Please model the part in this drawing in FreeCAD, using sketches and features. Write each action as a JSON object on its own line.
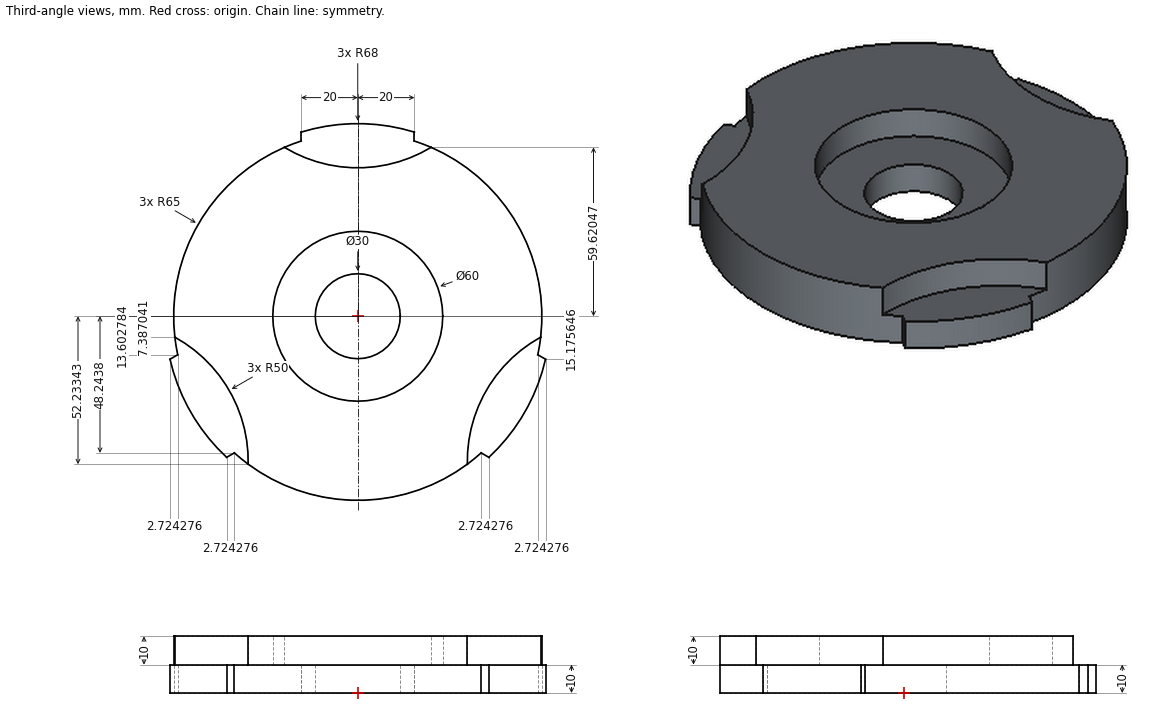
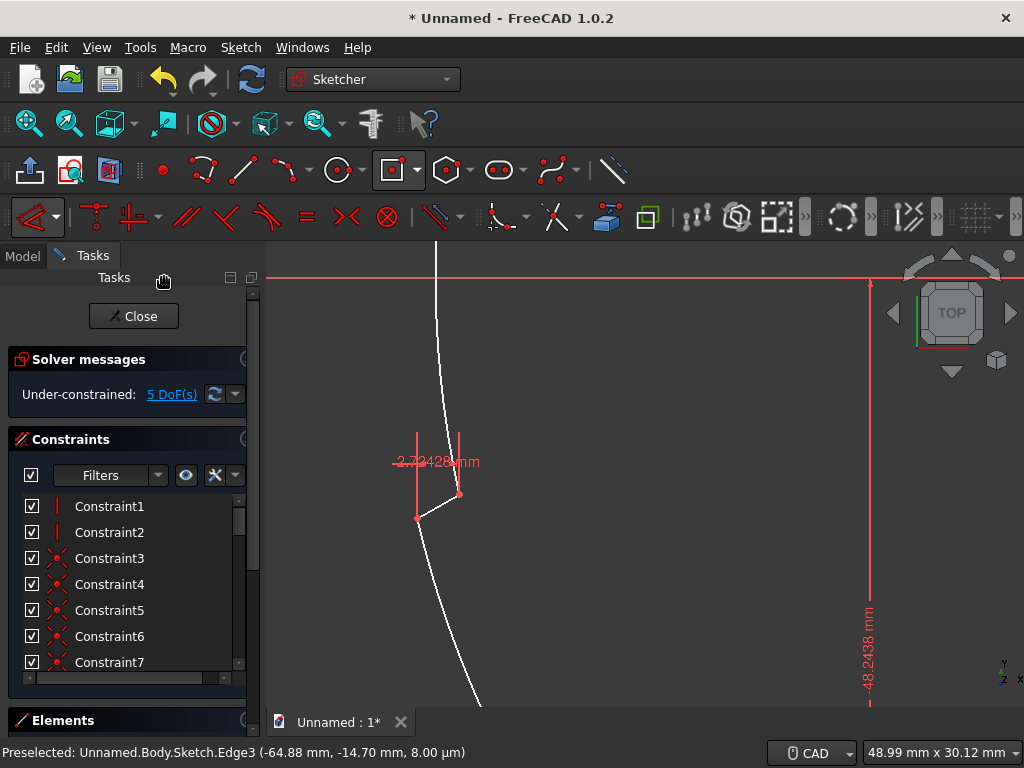
{"action": "scroll", "coordinate": [441, 508], "scroll_direction": "down", "scroll_amount": 10}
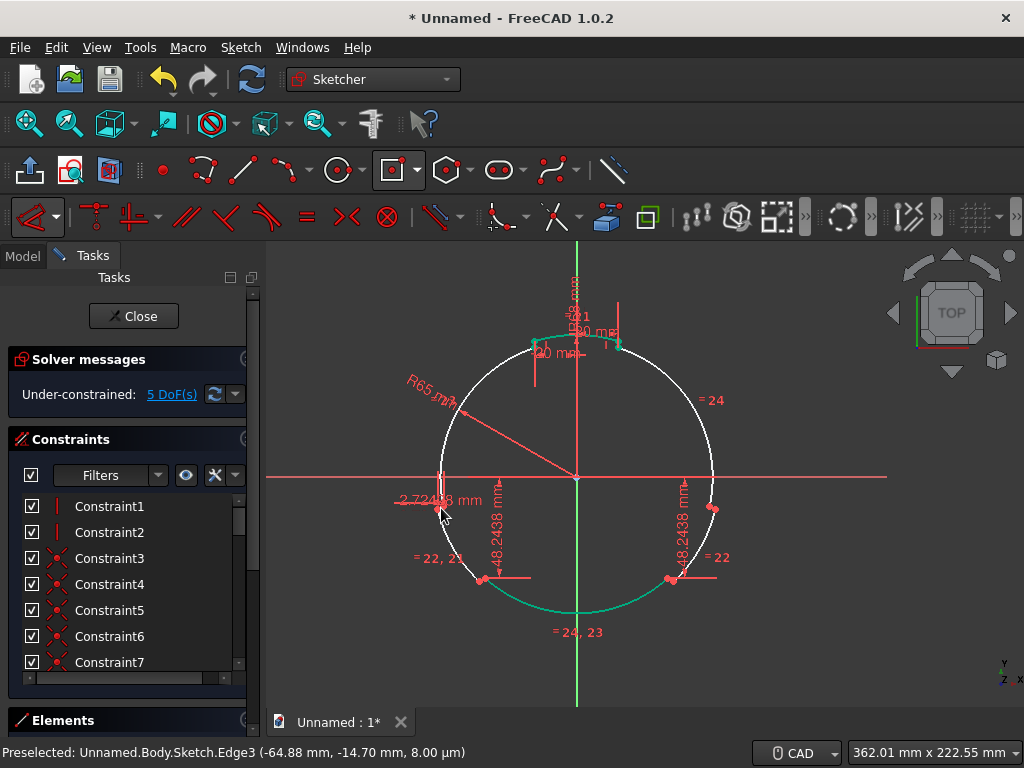
{"action": "scroll", "coordinate": [481, 581], "scroll_direction": "up", "scroll_amount": 10}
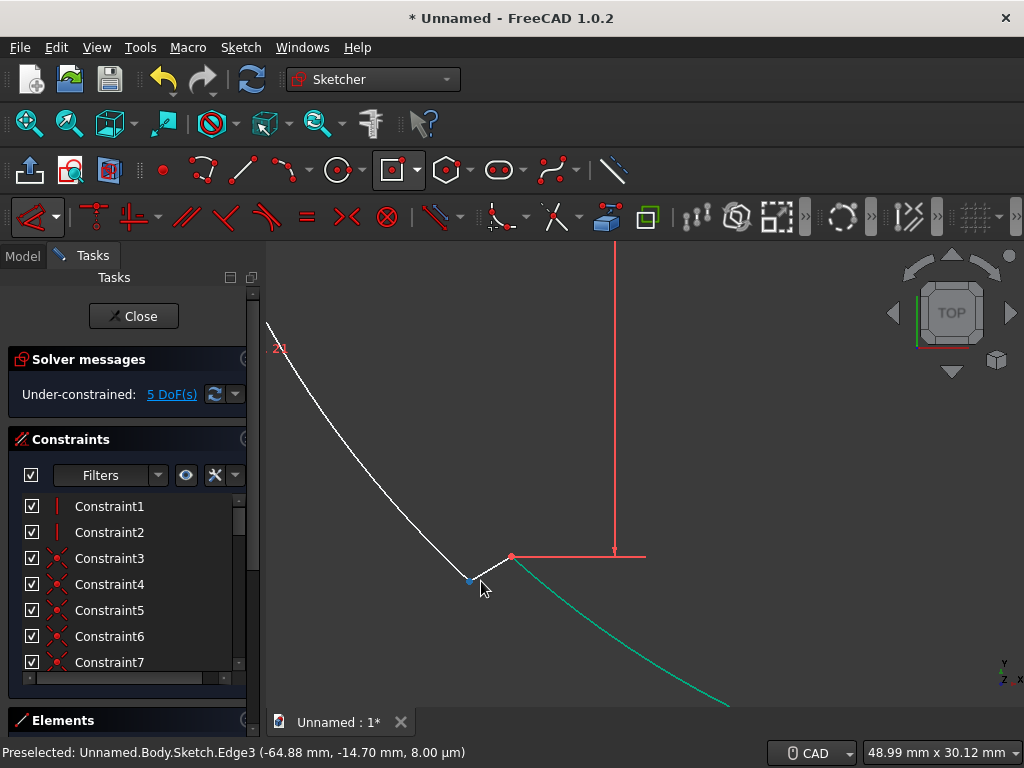
{"action": "left_click", "coordinate": [482, 574]}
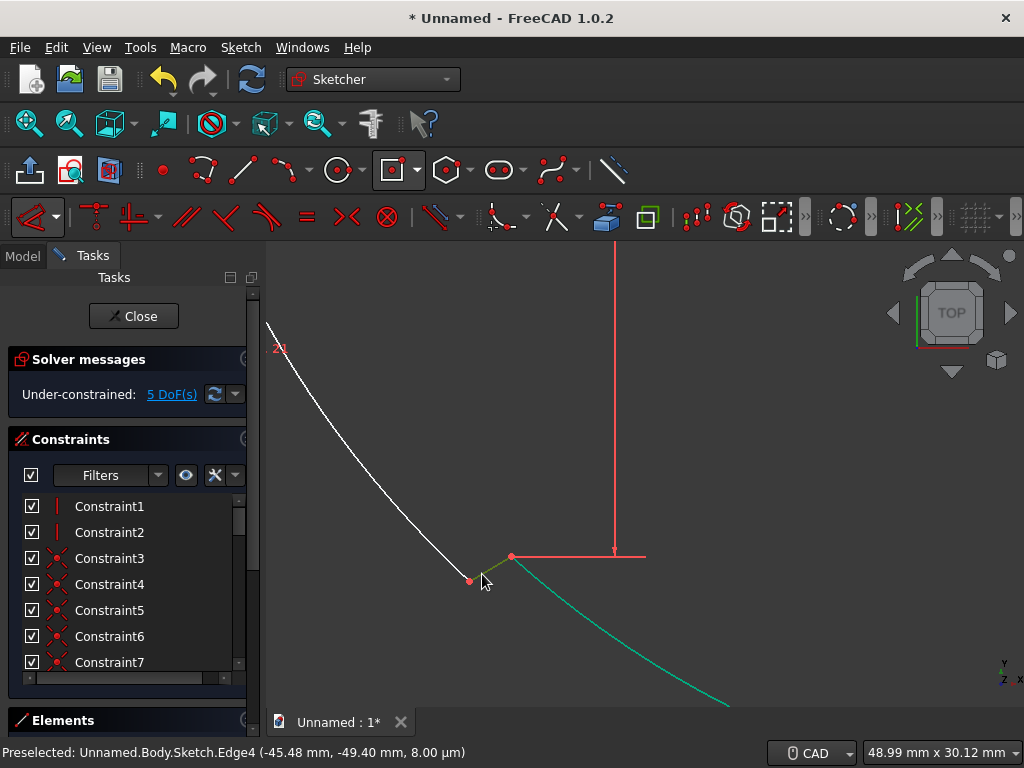
{"action": "key", "text": "l"}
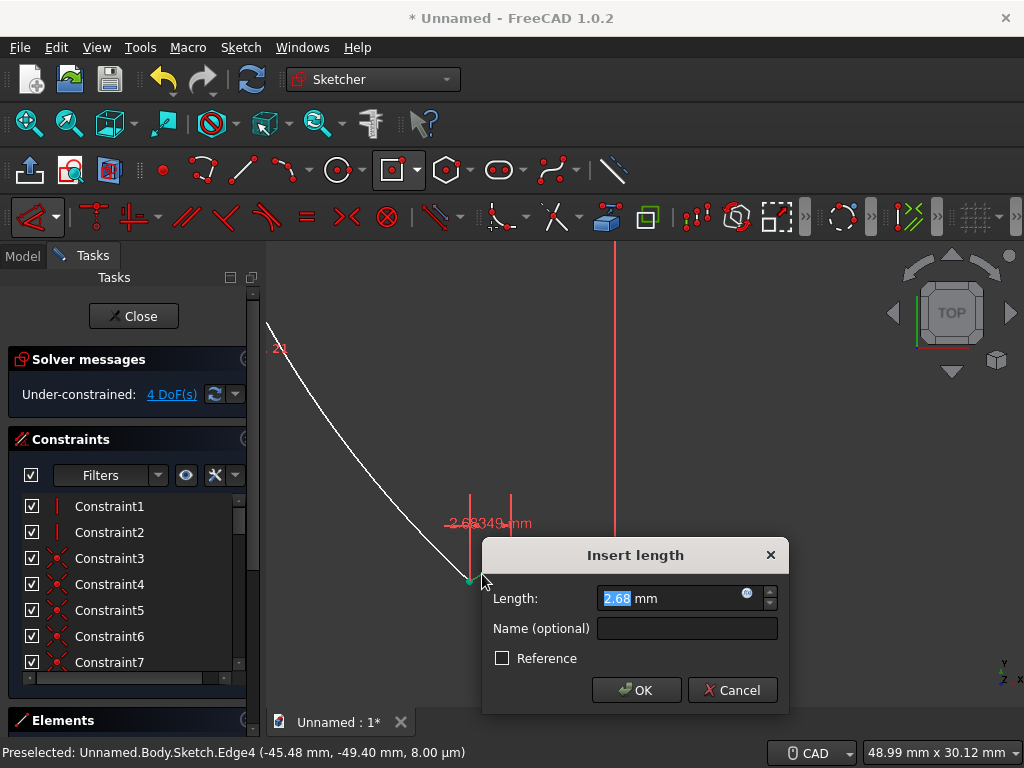
{"action": "type", "text": "2.724276"}
{"action": "key", "text": "Return"}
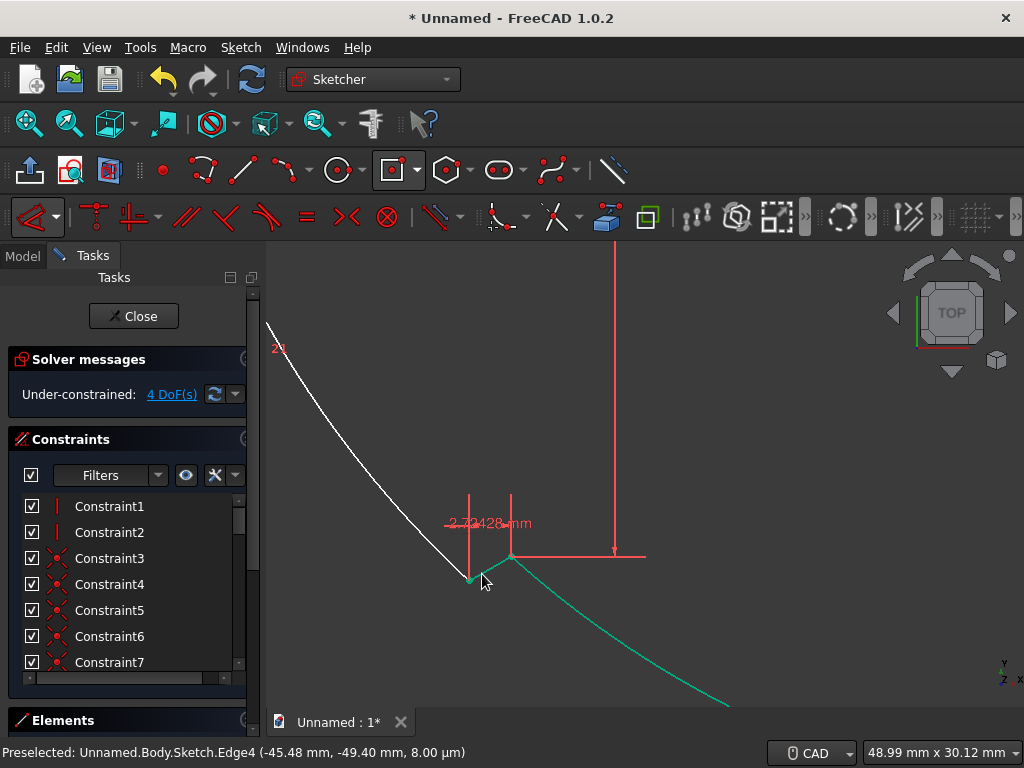
{"action": "scroll", "coordinate": [481, 582], "scroll_direction": "down", "scroll_amount": 10}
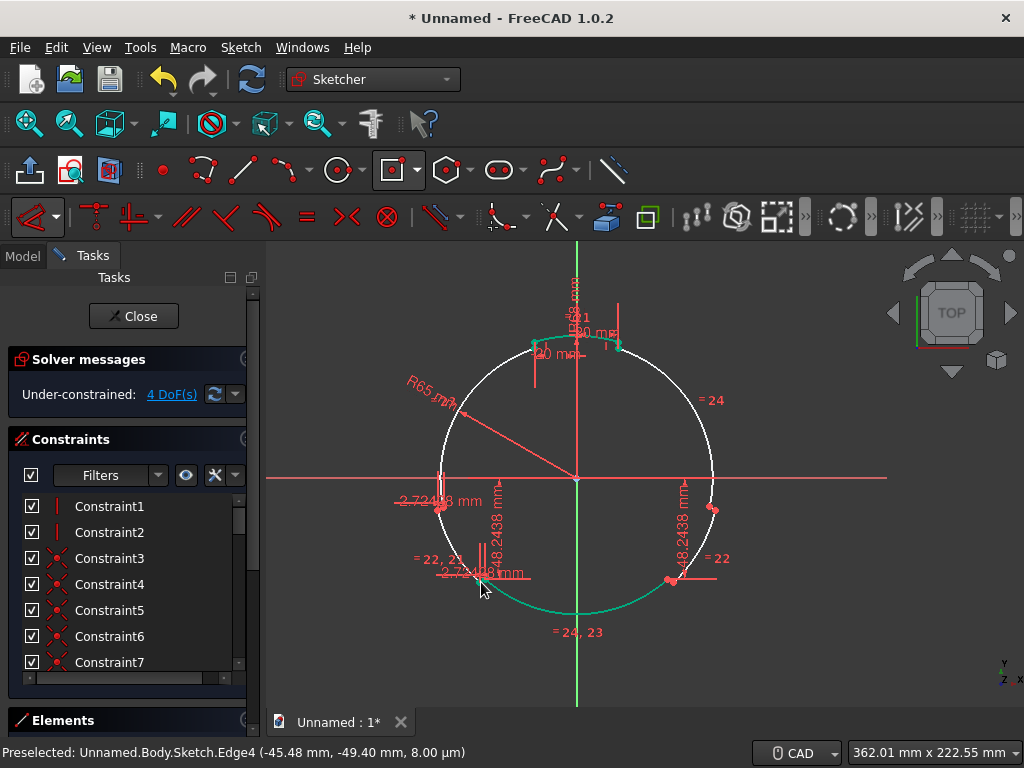
{"action": "scroll", "coordinate": [670, 580], "scroll_direction": "up", "scroll_amount": 10}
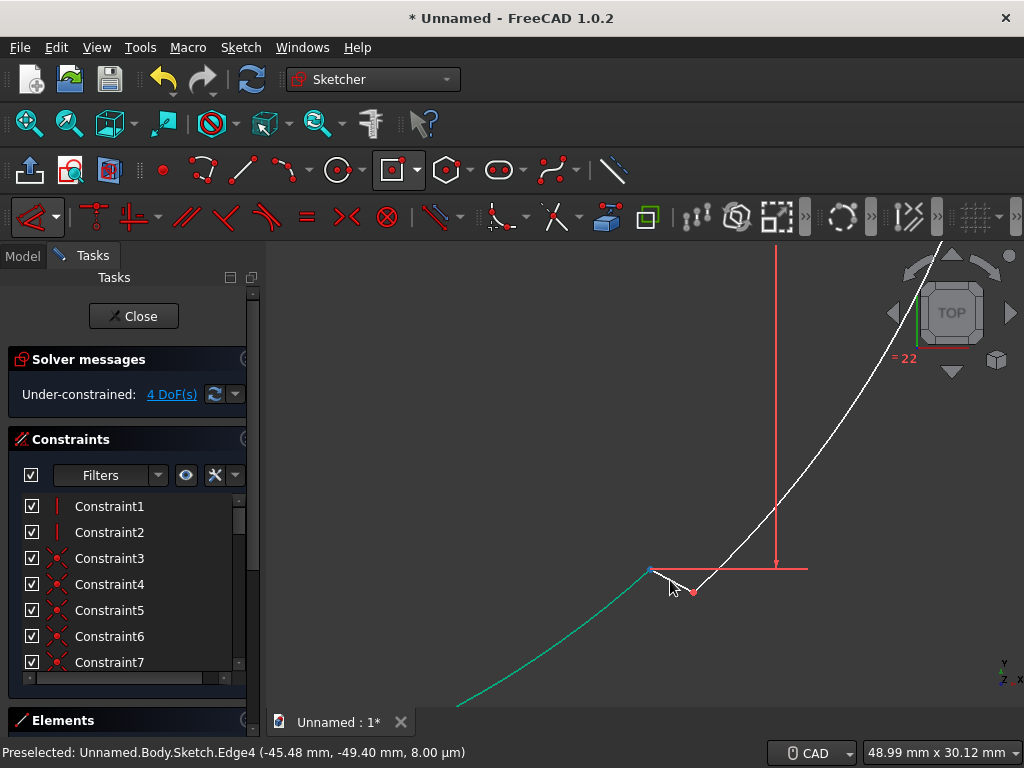
{"action": "left_click", "coordinate": [663, 576]}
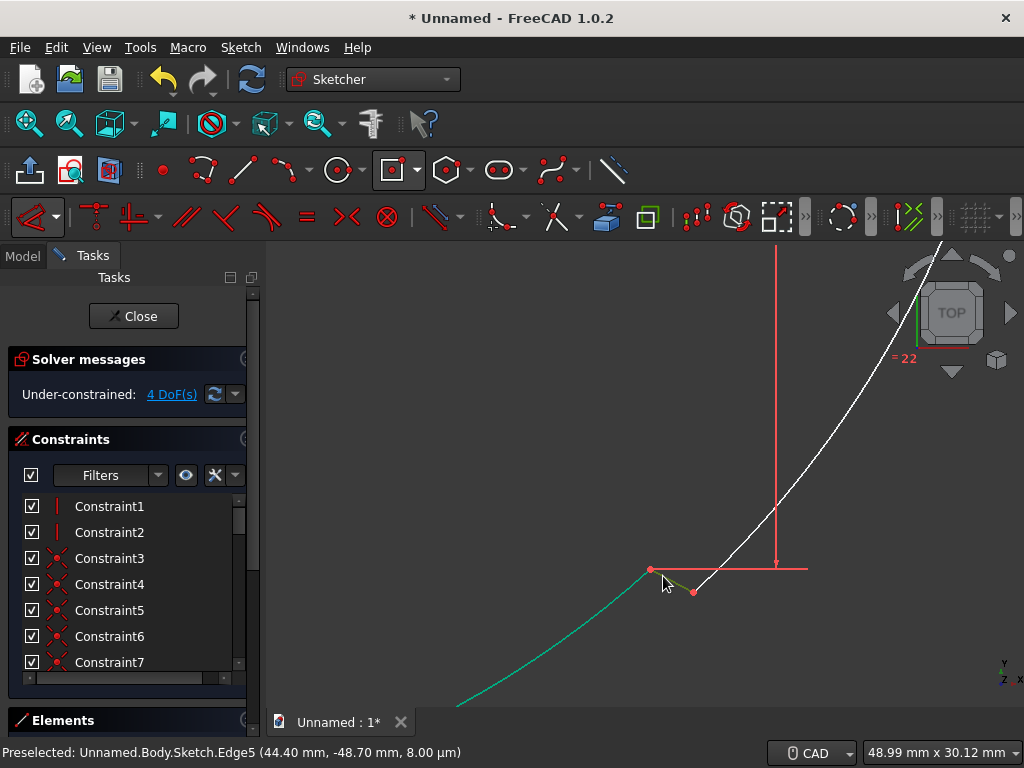
{"action": "key", "text": "l"}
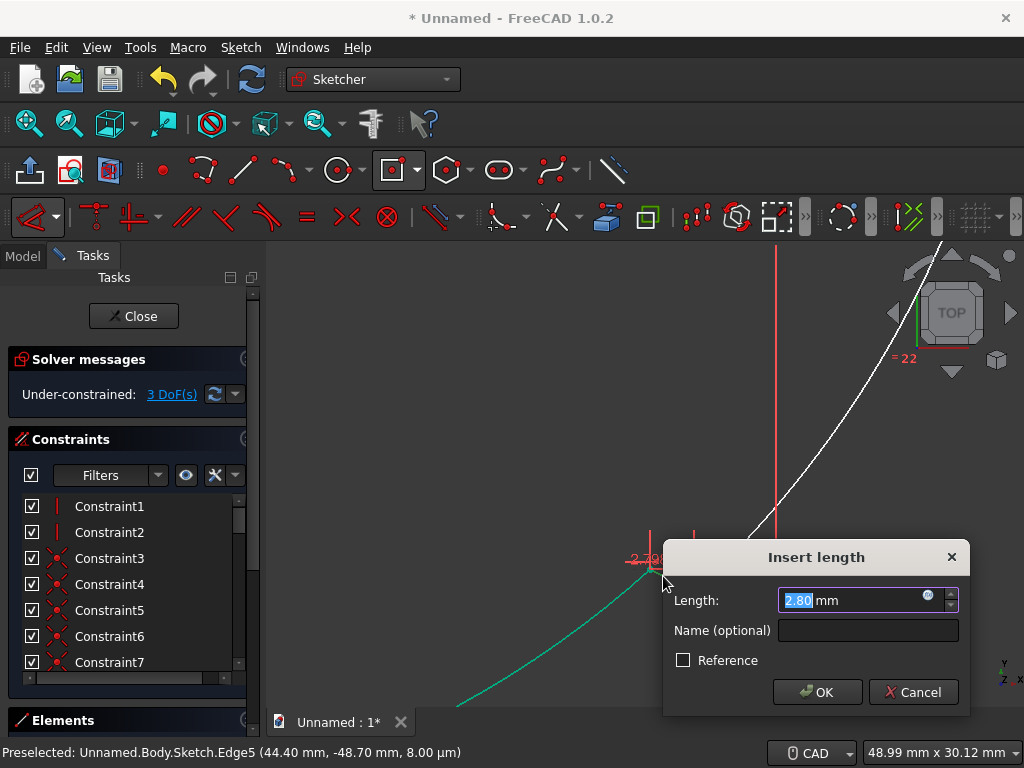
{"action": "type", "text": "2.724276"}
{"action": "key", "text": "Return"}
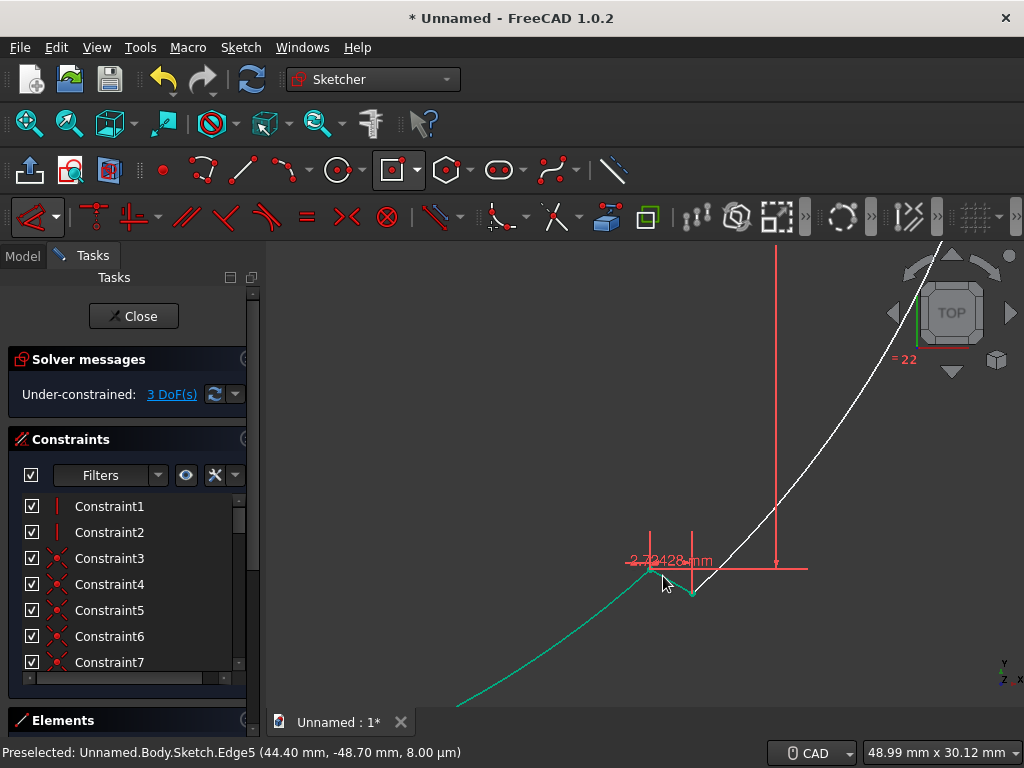
{"action": "scroll", "coordinate": [670, 580], "scroll_direction": "down", "scroll_amount": 10}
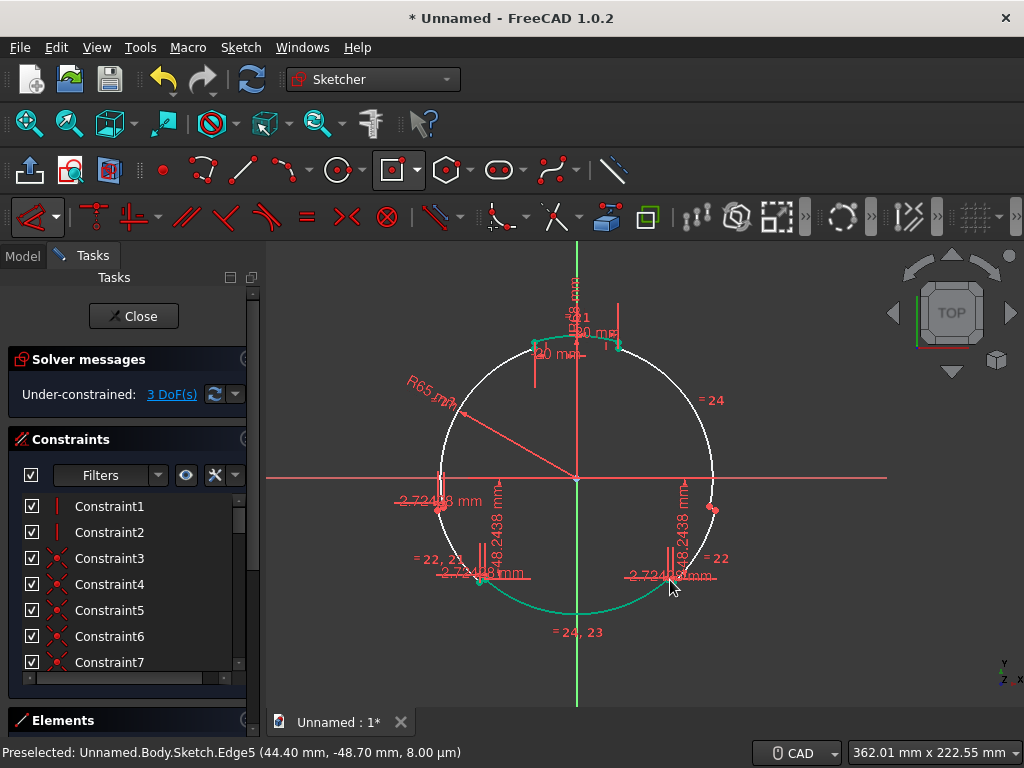
{"action": "scroll", "coordinate": [714, 509], "scroll_direction": "up", "scroll_amount": 10}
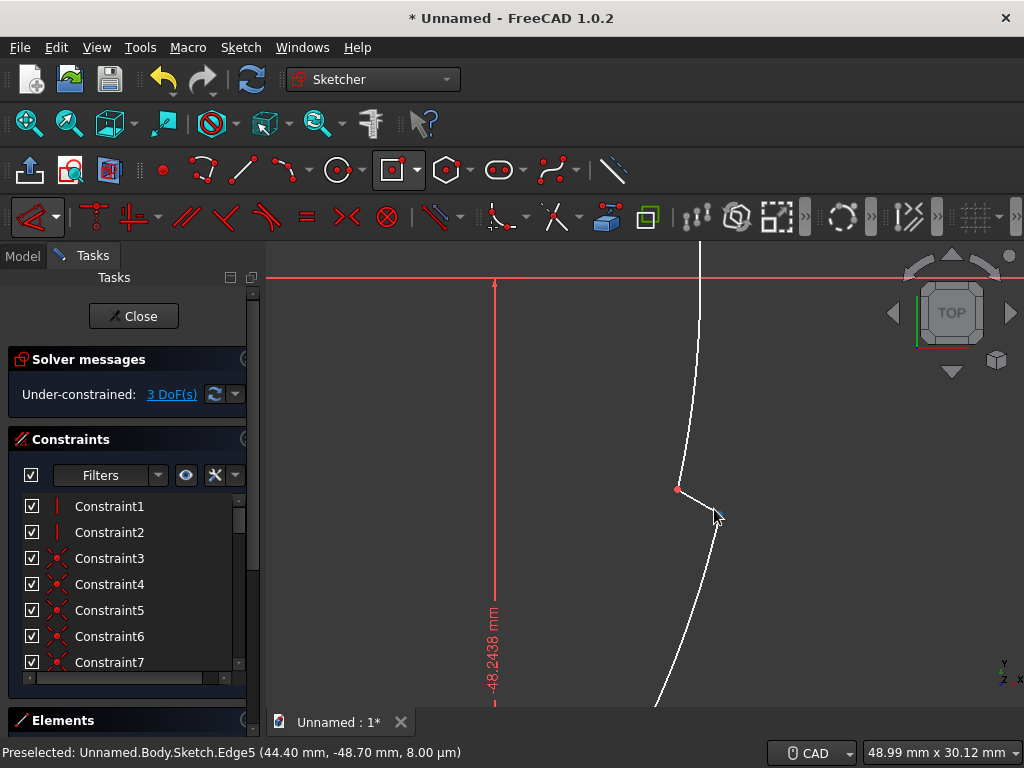
{"action": "left_click", "coordinate": [707, 507]}